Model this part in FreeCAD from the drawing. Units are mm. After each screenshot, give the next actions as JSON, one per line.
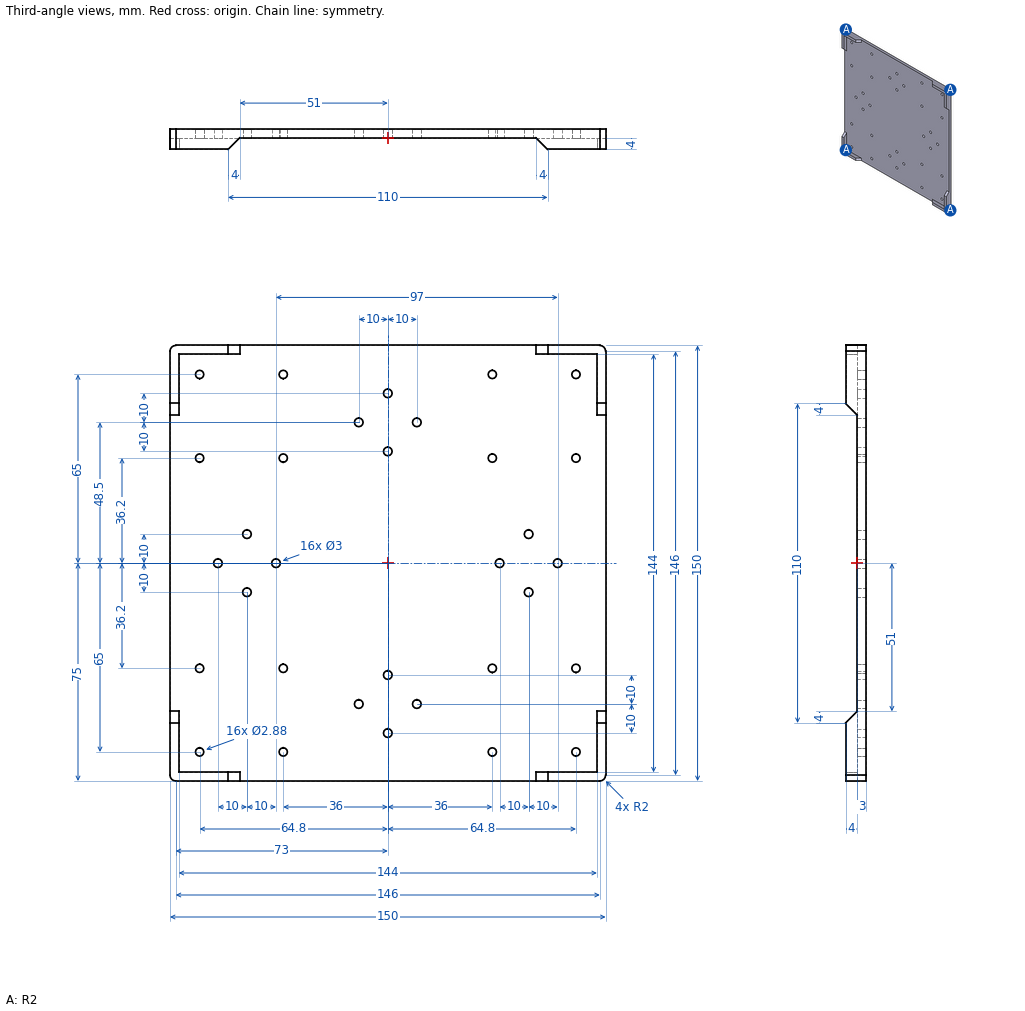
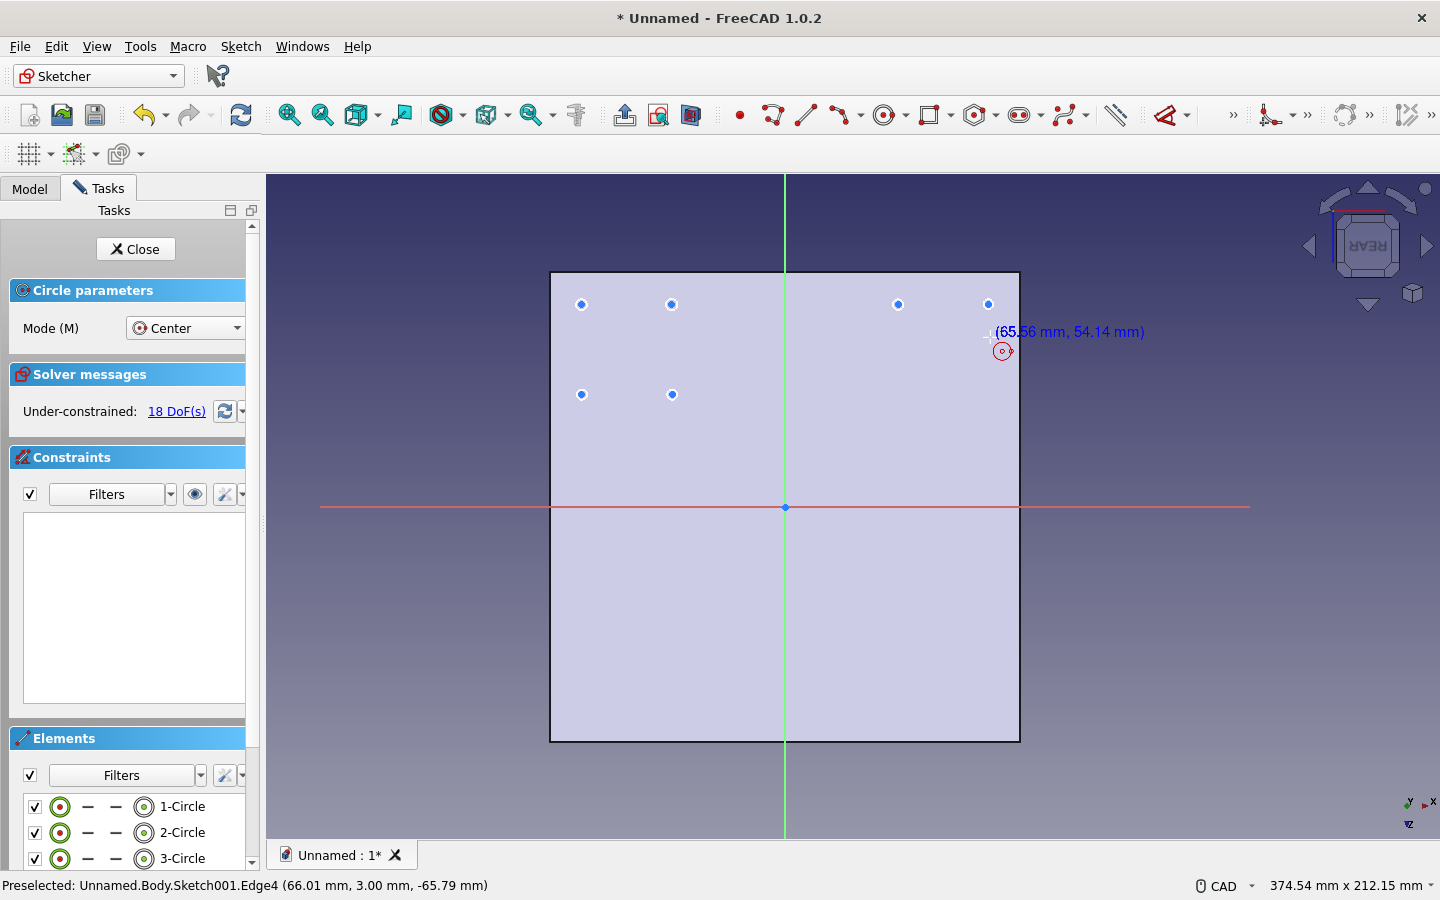
{"action": "left_click", "coordinate": [988, 394]}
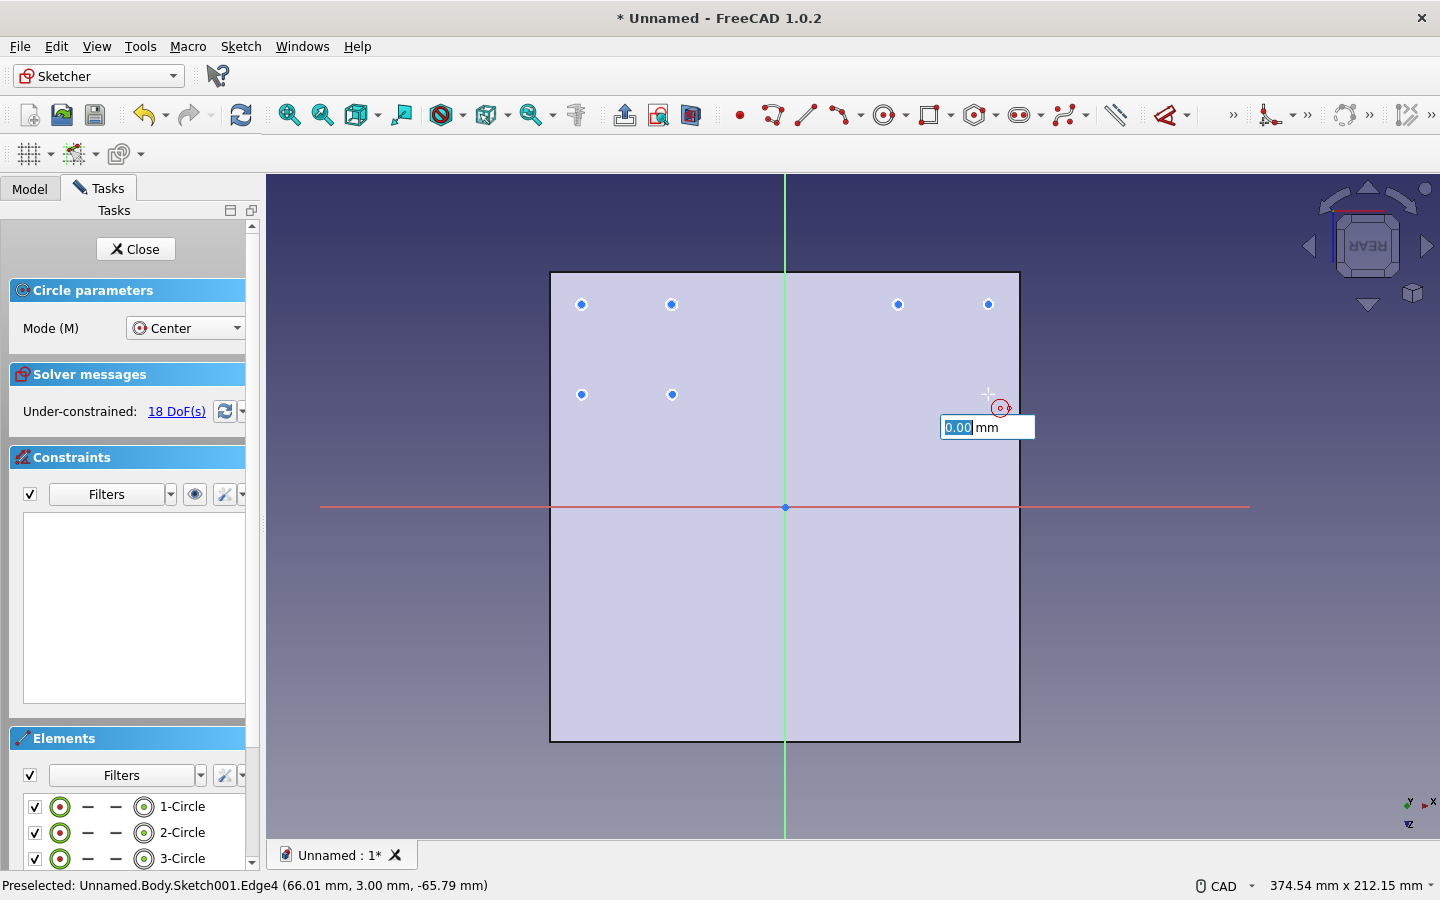
{"action": "scroll", "coordinate": [991, 390], "scroll_direction": "up", "scroll_amount": 7}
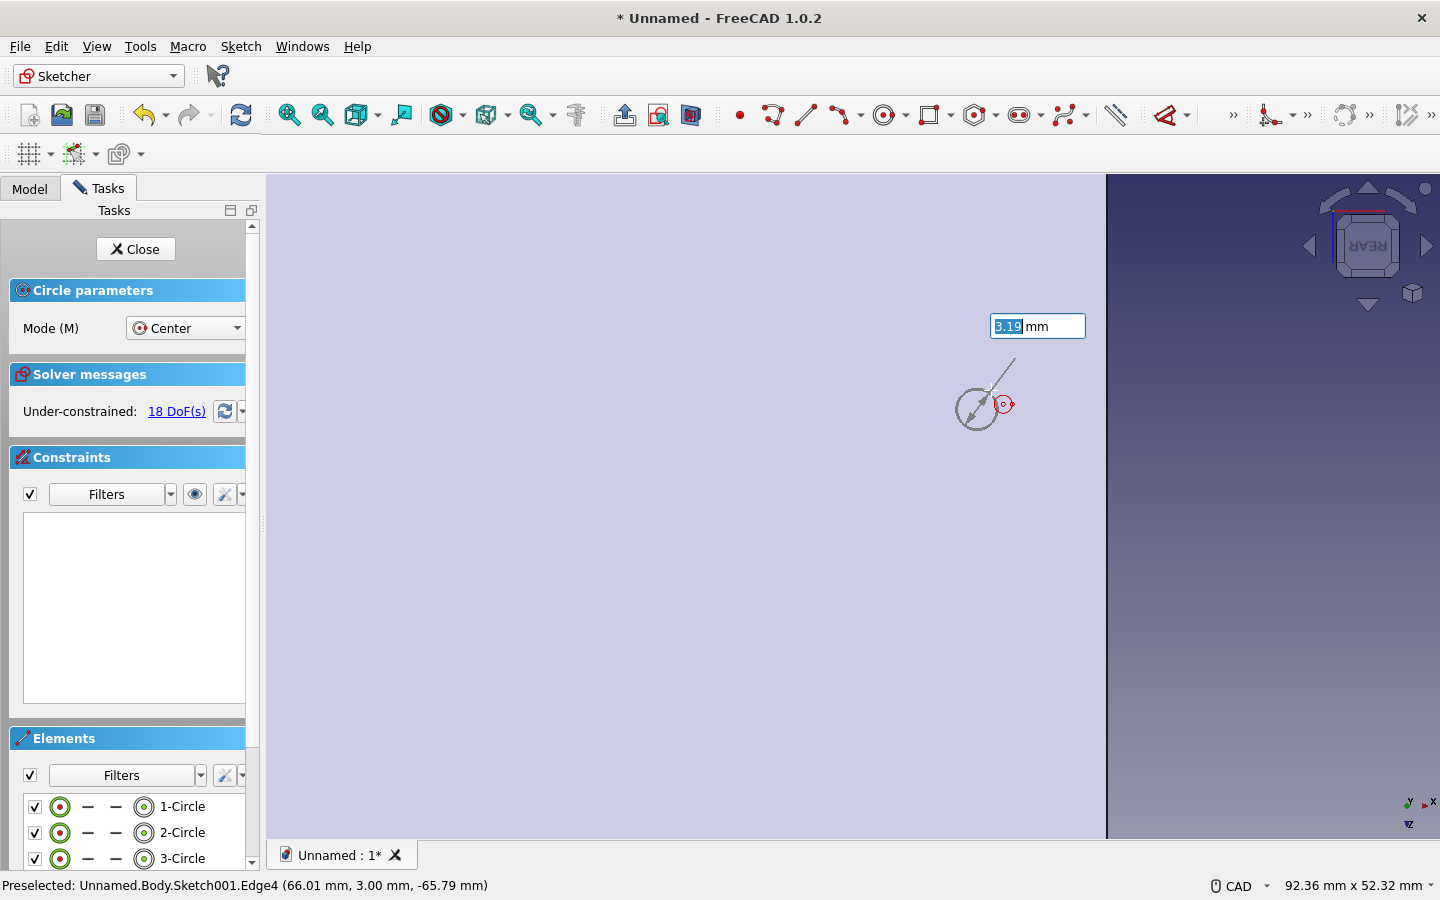
{"action": "left_click", "coordinate": [990, 391]}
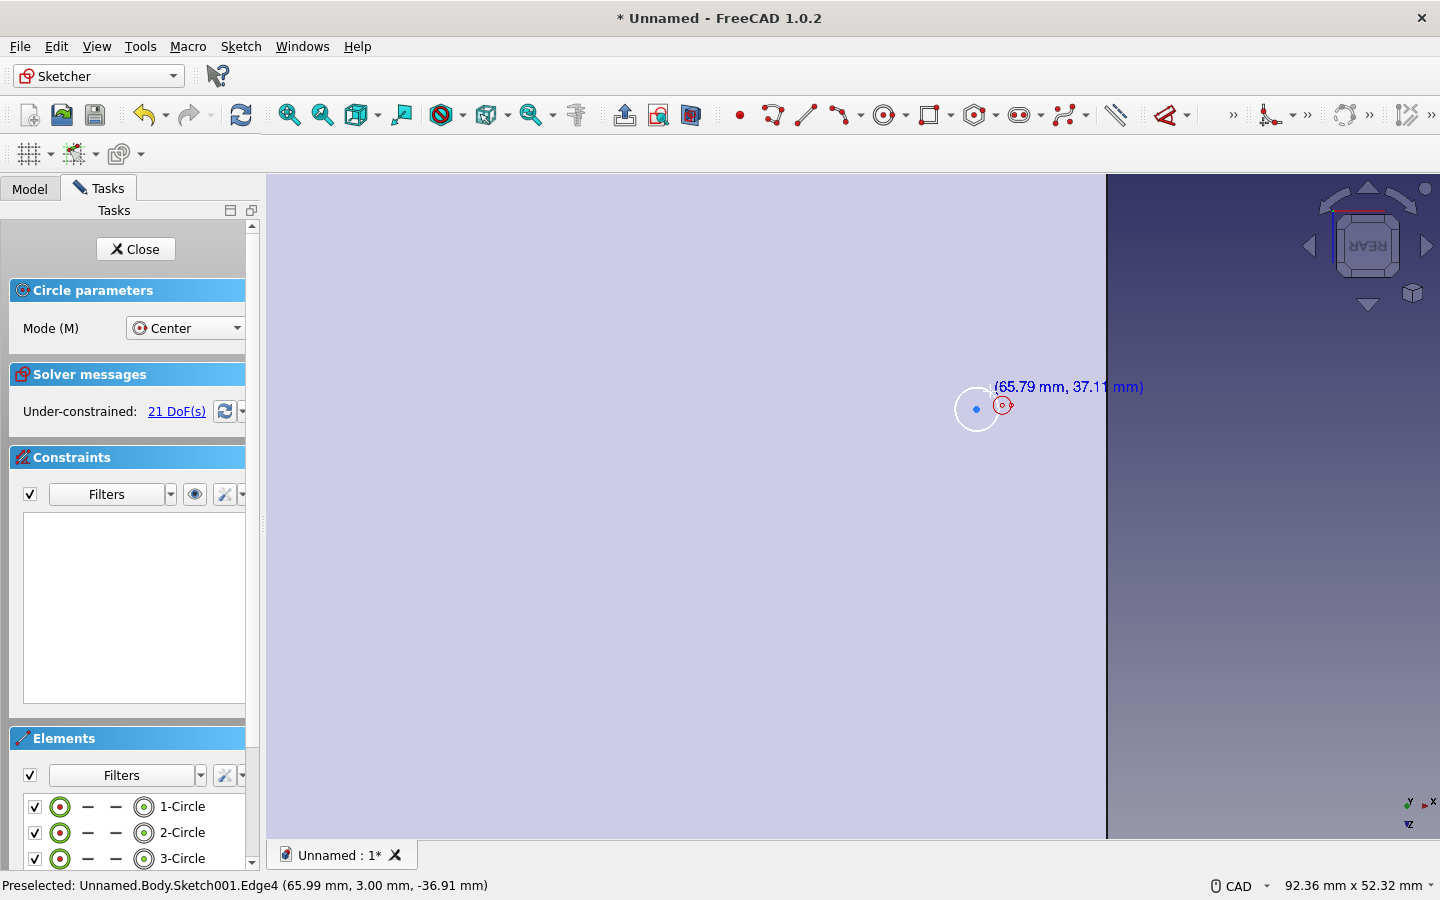
{"action": "scroll", "coordinate": [611, 404], "scroll_direction": "up", "scroll_amount": 2}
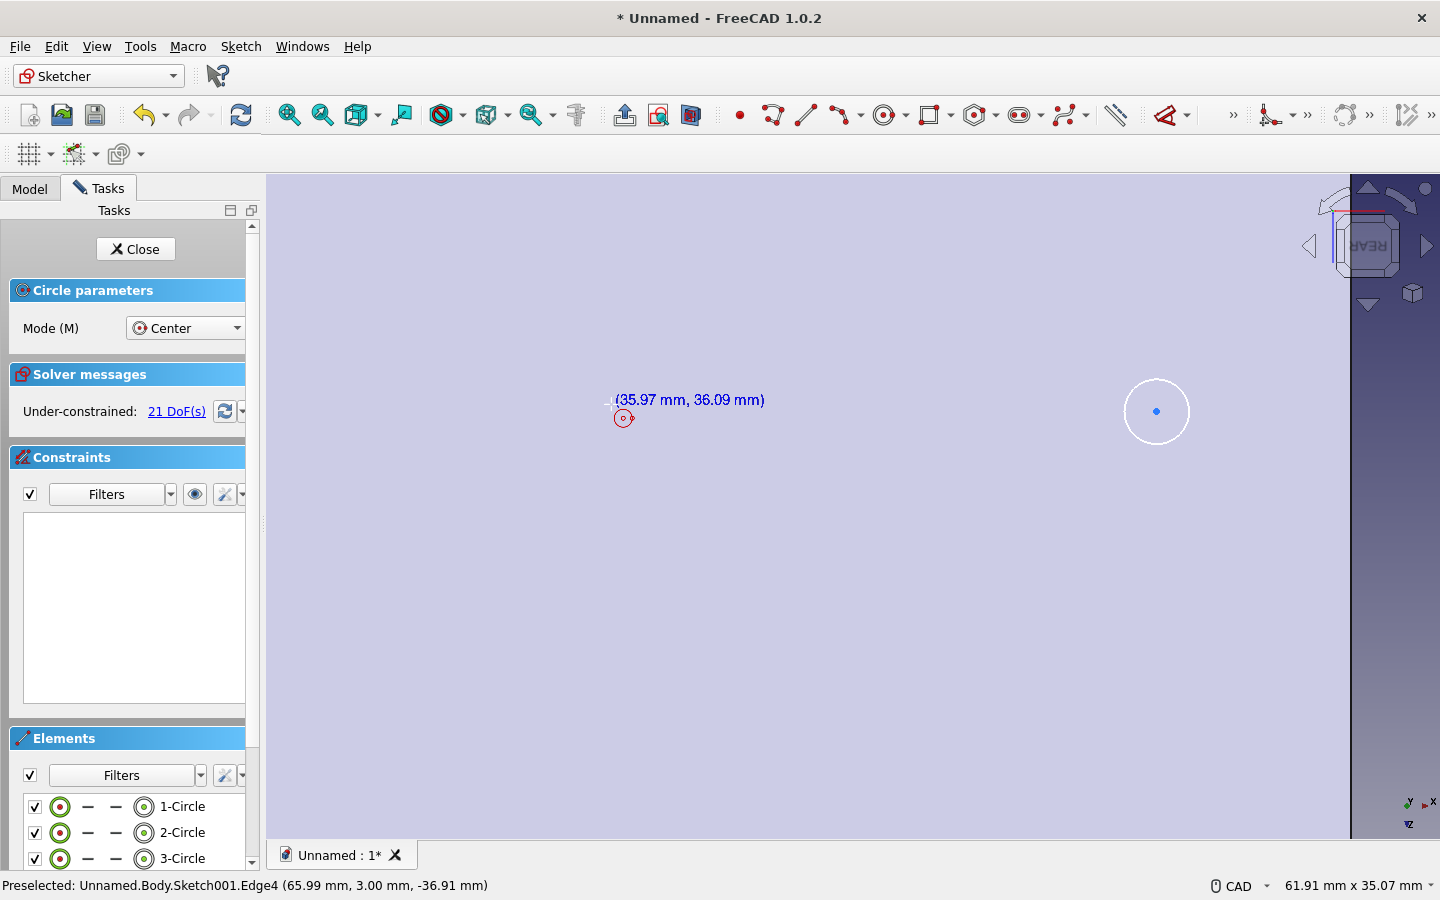
{"action": "scroll", "coordinate": [954, 391], "scroll_direction": "down", "scroll_amount": 9}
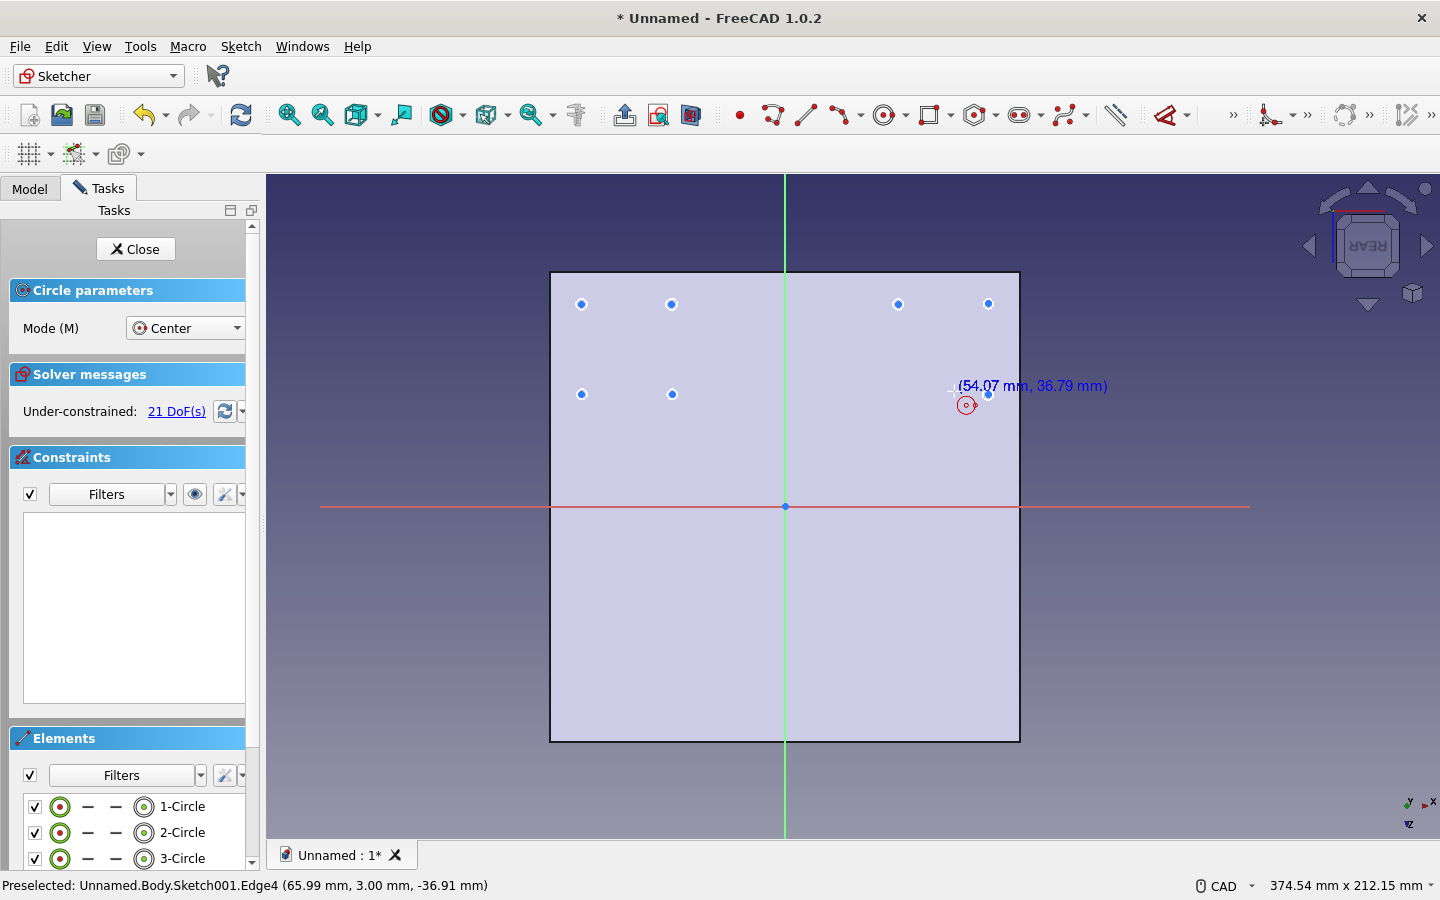
{"action": "left_click", "coordinate": [898, 393]}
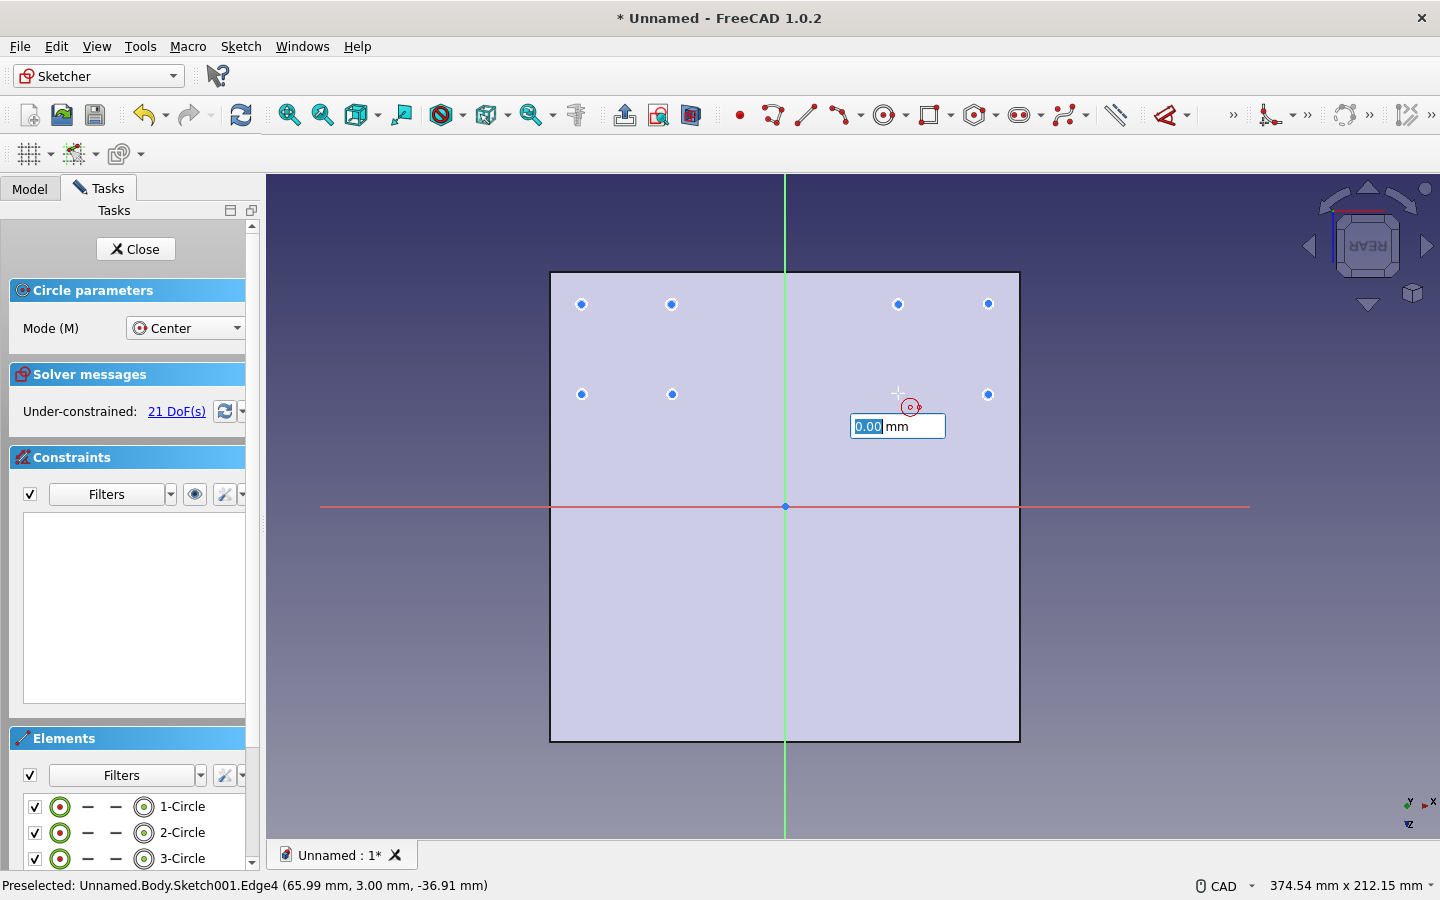
{"action": "scroll", "coordinate": [901, 390], "scroll_direction": "up", "scroll_amount": 7}